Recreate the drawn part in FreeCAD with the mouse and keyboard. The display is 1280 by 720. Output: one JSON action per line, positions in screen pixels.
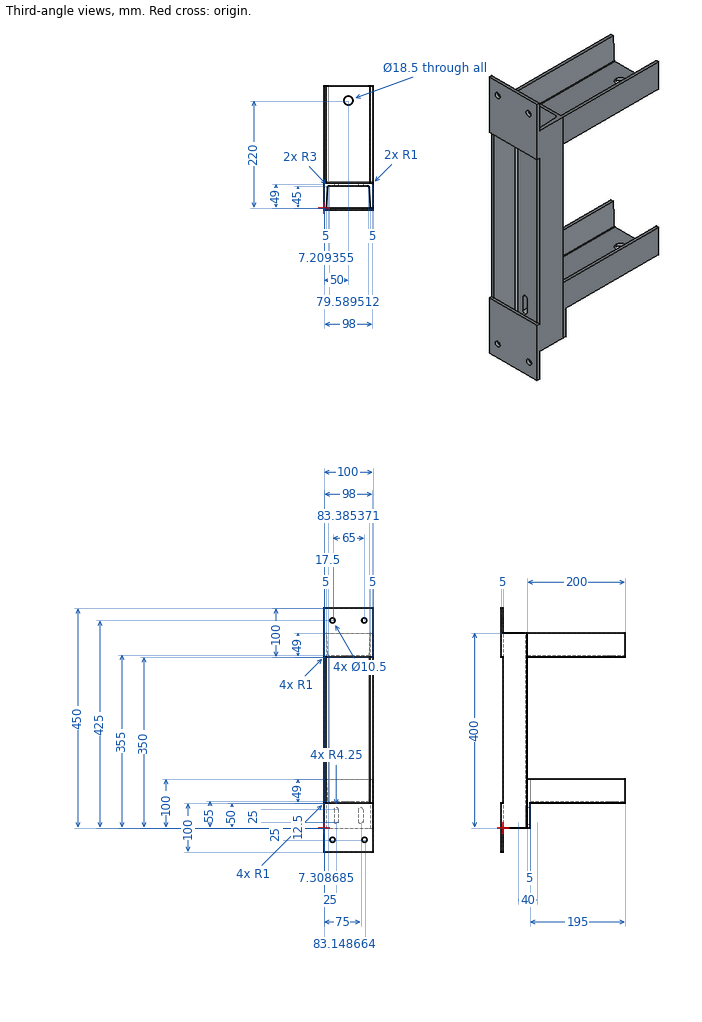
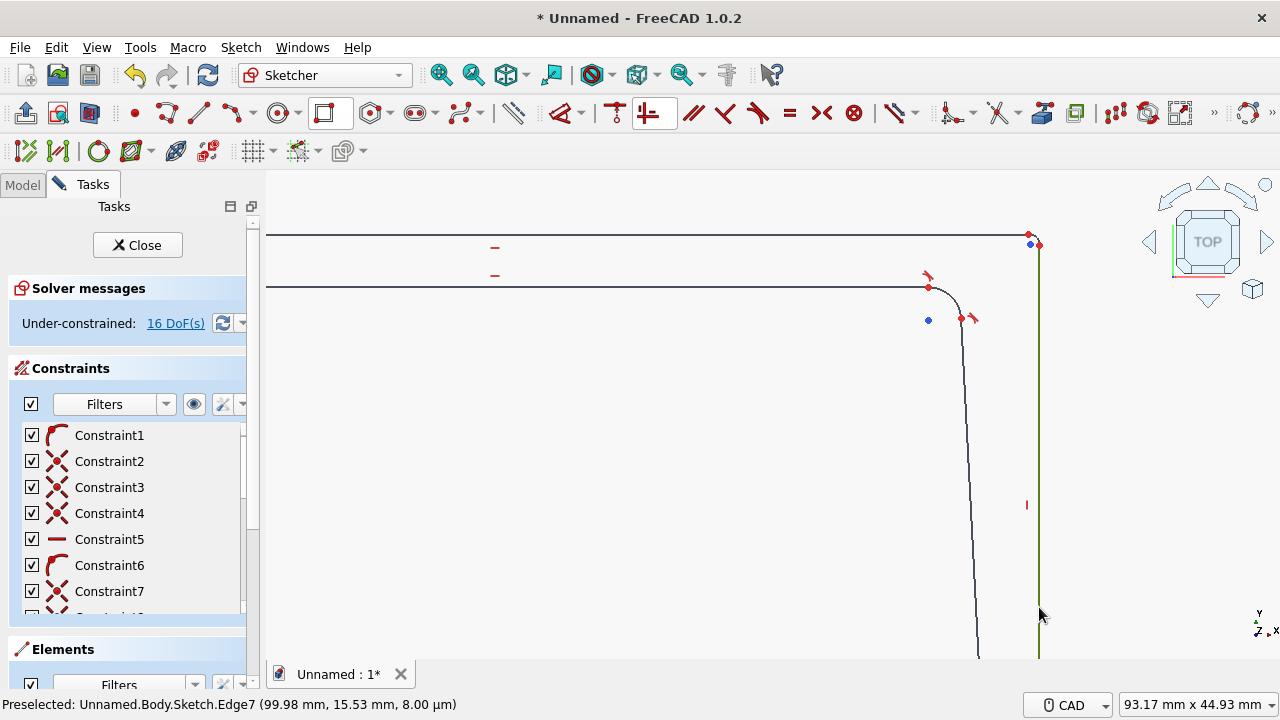
{"action": "scroll", "coordinate": [1037, 237], "scroll_direction": "up", "scroll_amount": 3}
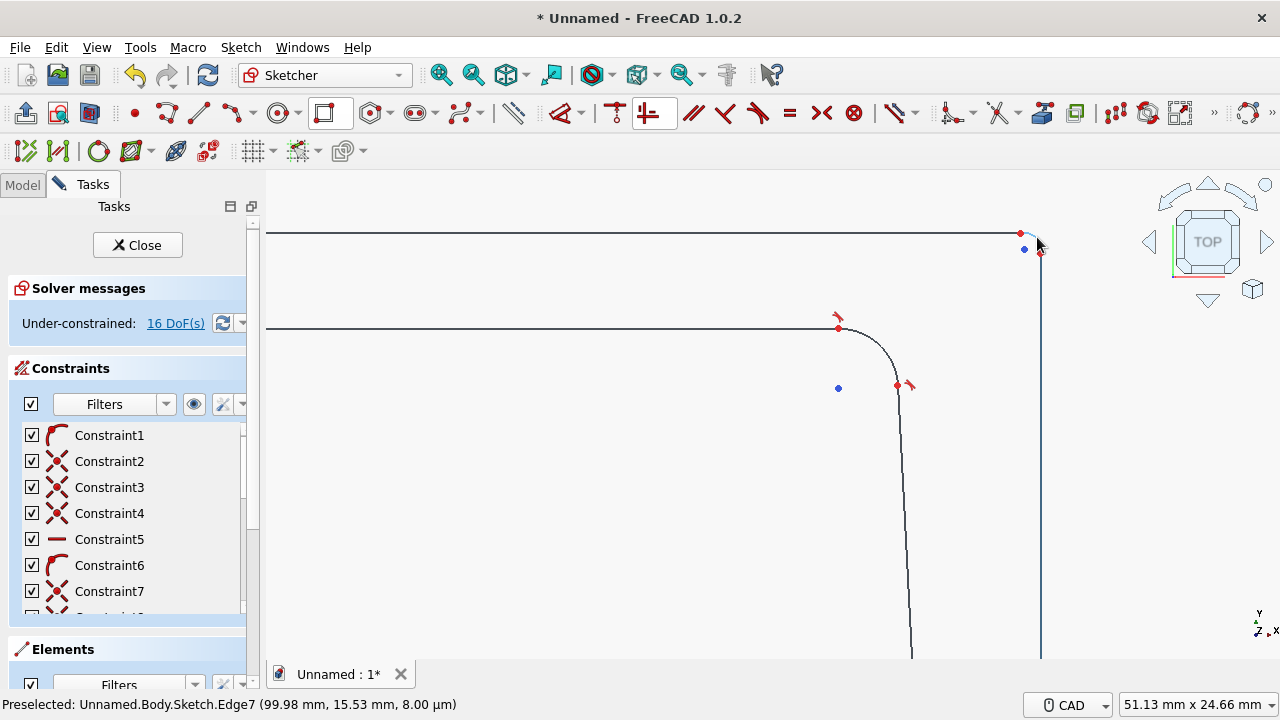
{"action": "left_click", "coordinate": [1036, 238]}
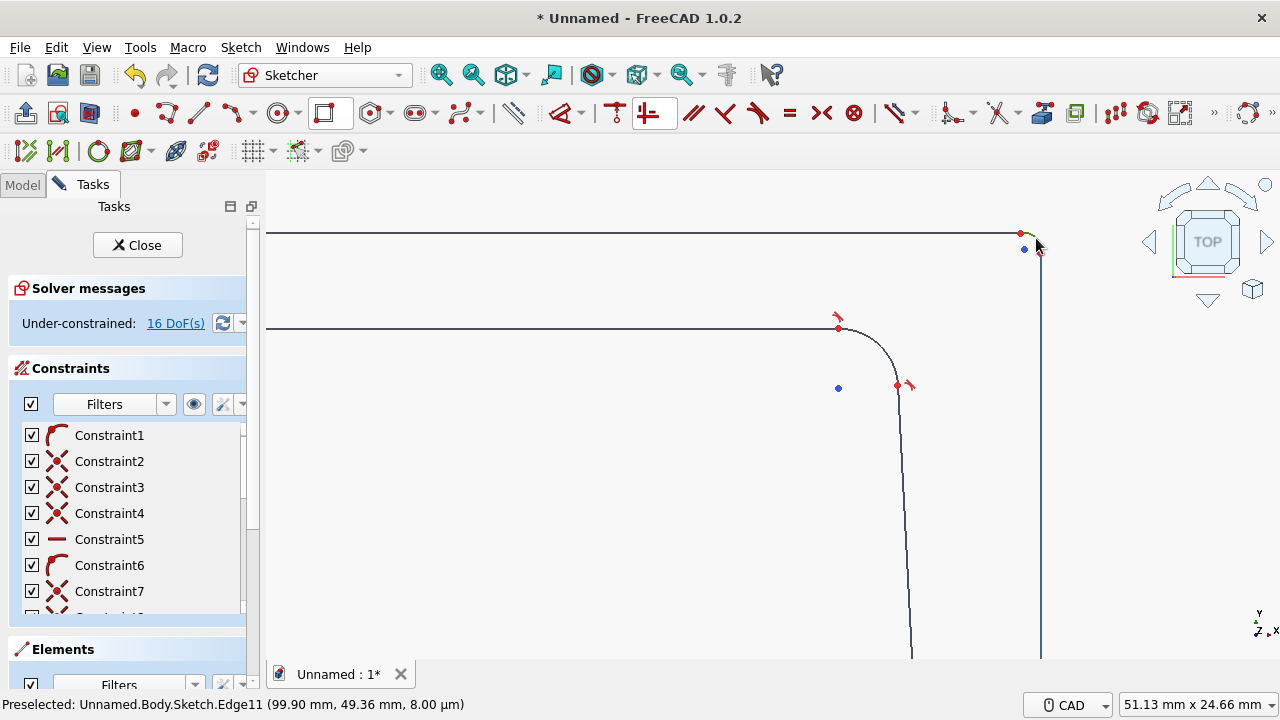
{"action": "left_click", "coordinate": [758, 114]}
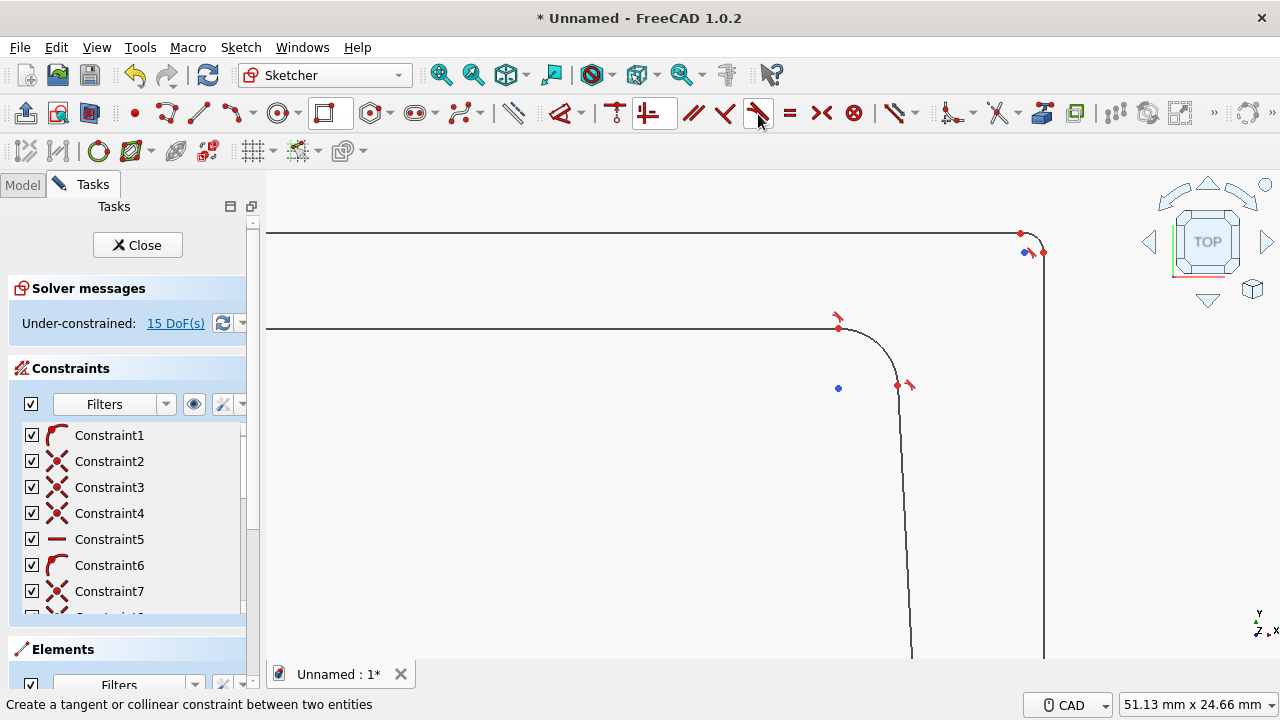
{"action": "left_click", "coordinate": [437, 233]}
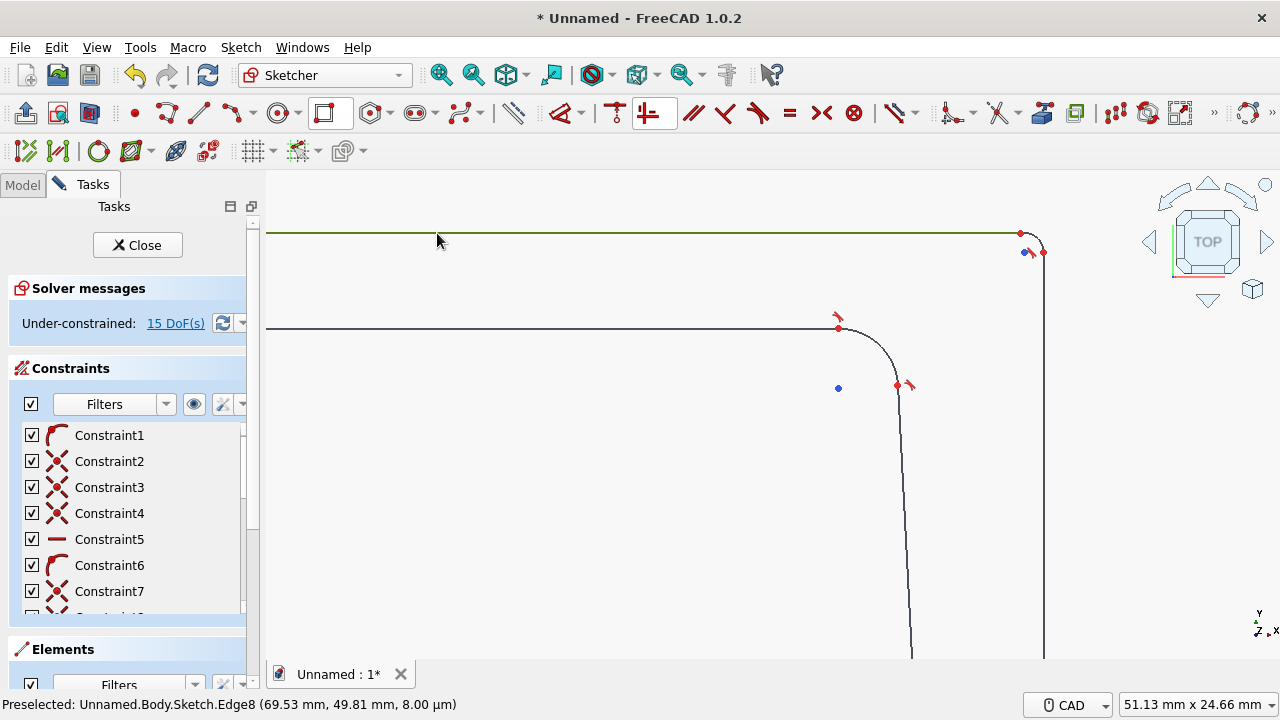
{"action": "scroll", "coordinate": [1041, 242], "scroll_direction": "up", "scroll_amount": 2}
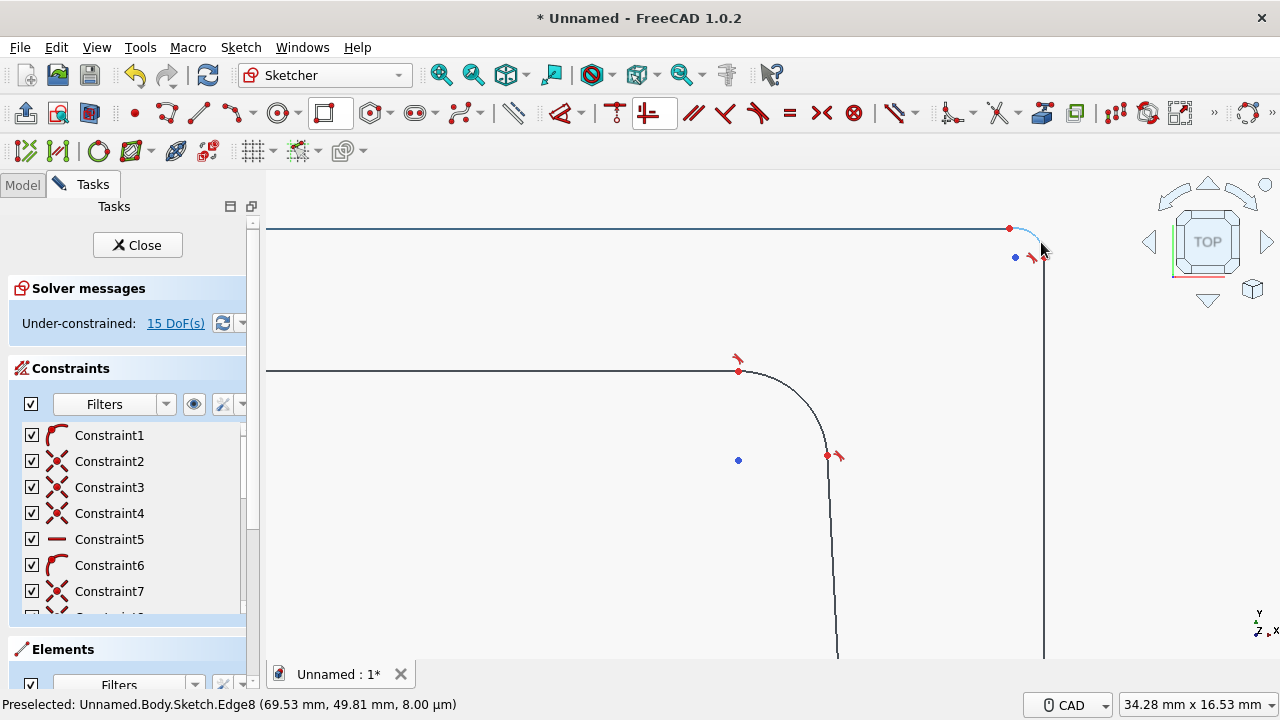
{"action": "left_click", "coordinate": [1040, 243]}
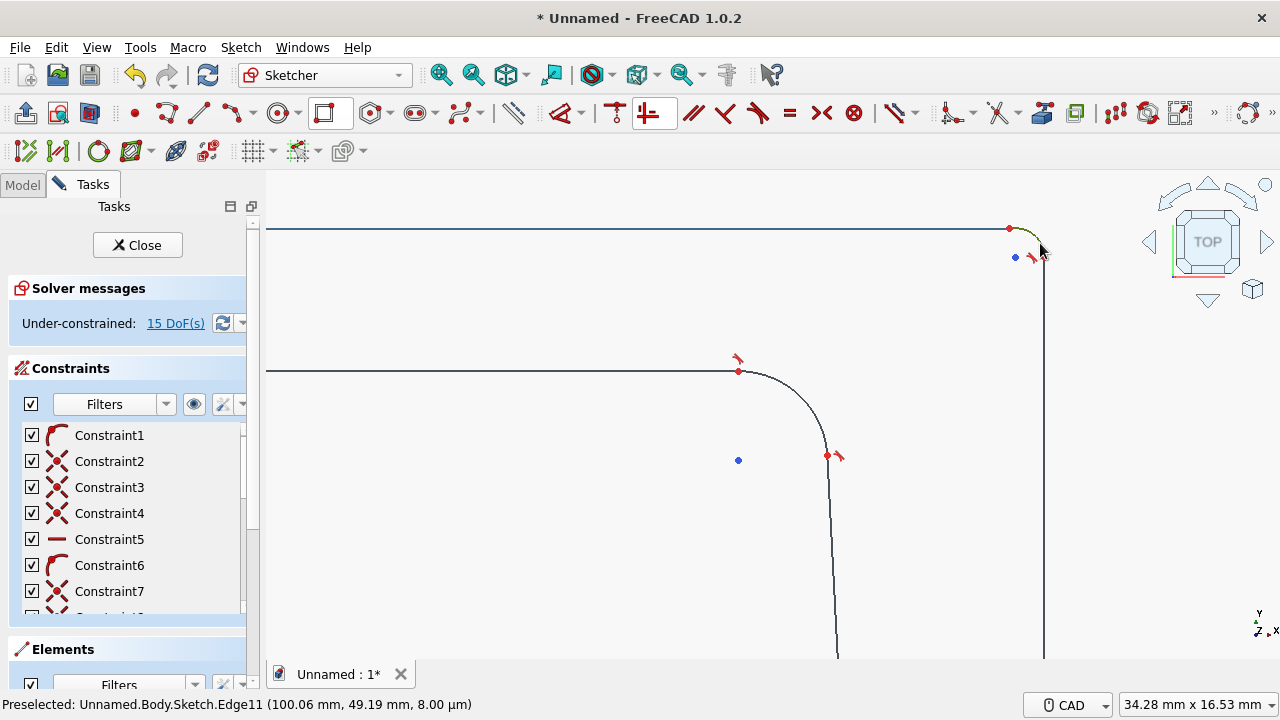
{"action": "left_click", "coordinate": [758, 114]}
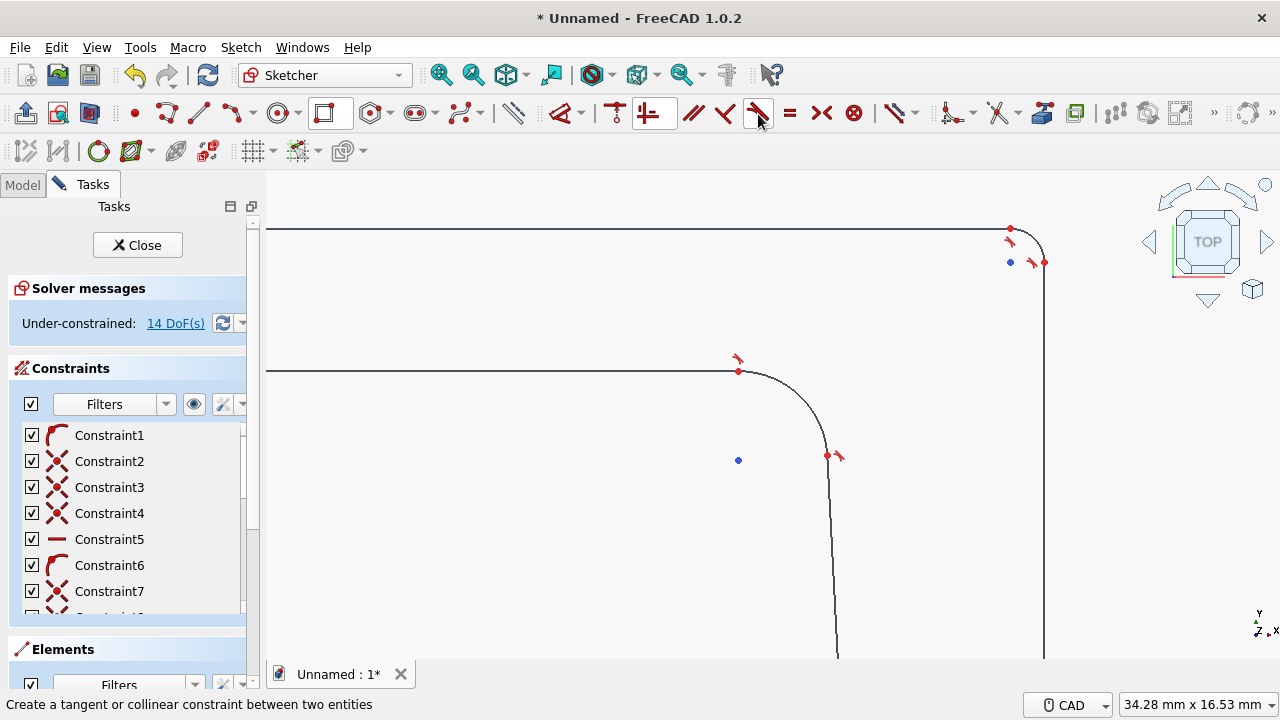
{"action": "scroll", "coordinate": [994, 276], "scroll_direction": "down", "scroll_amount": 8}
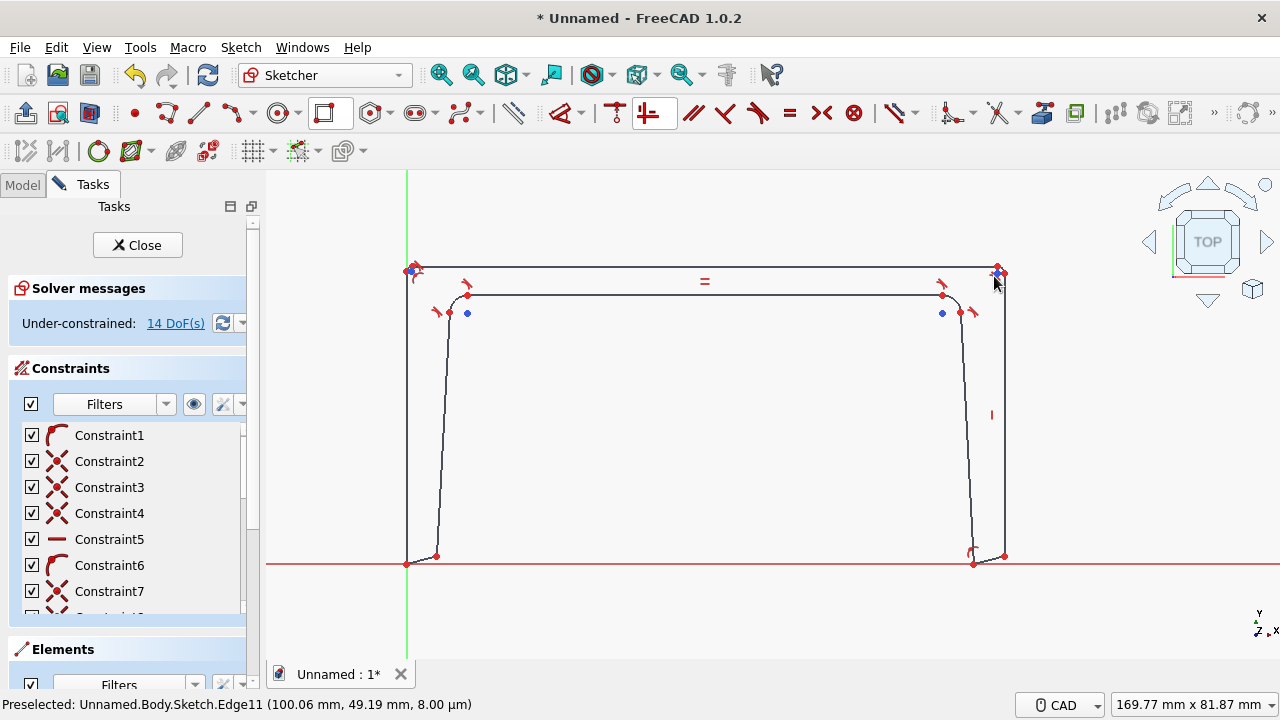
{"action": "left_click", "coordinate": [881, 267]}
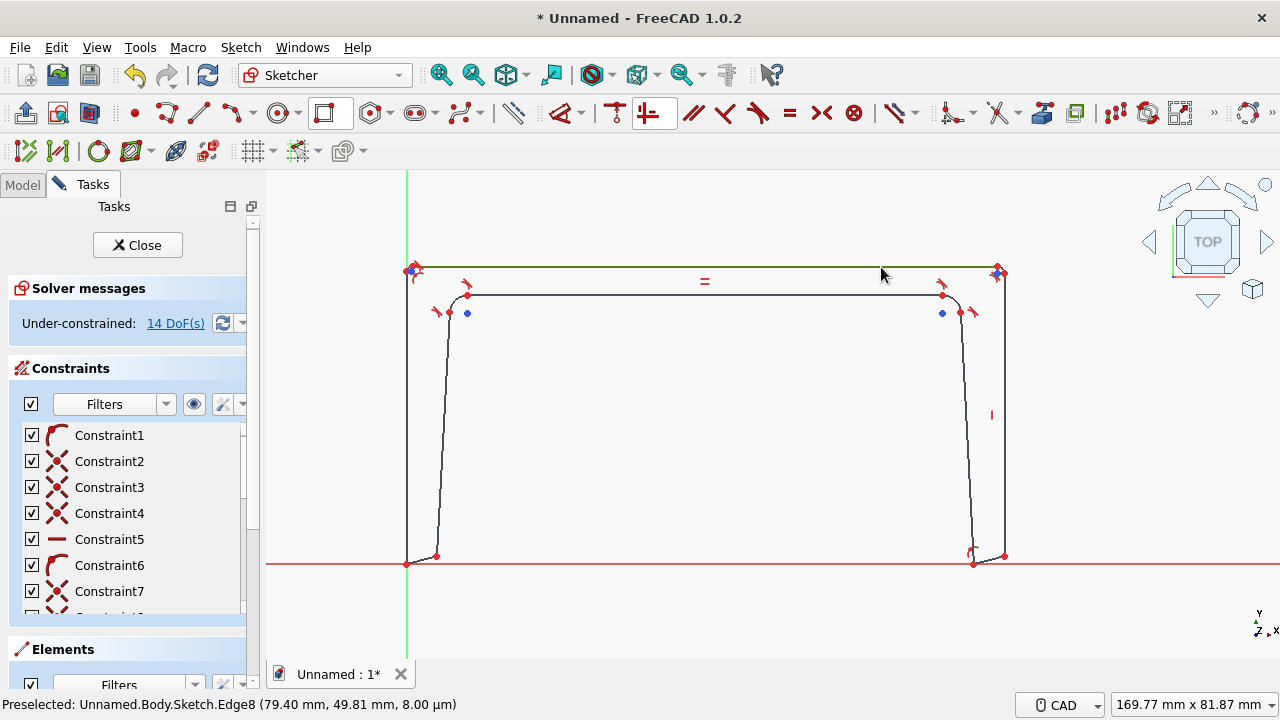
{"action": "scroll", "coordinate": [409, 268], "scroll_direction": "up", "scroll_amount": 6}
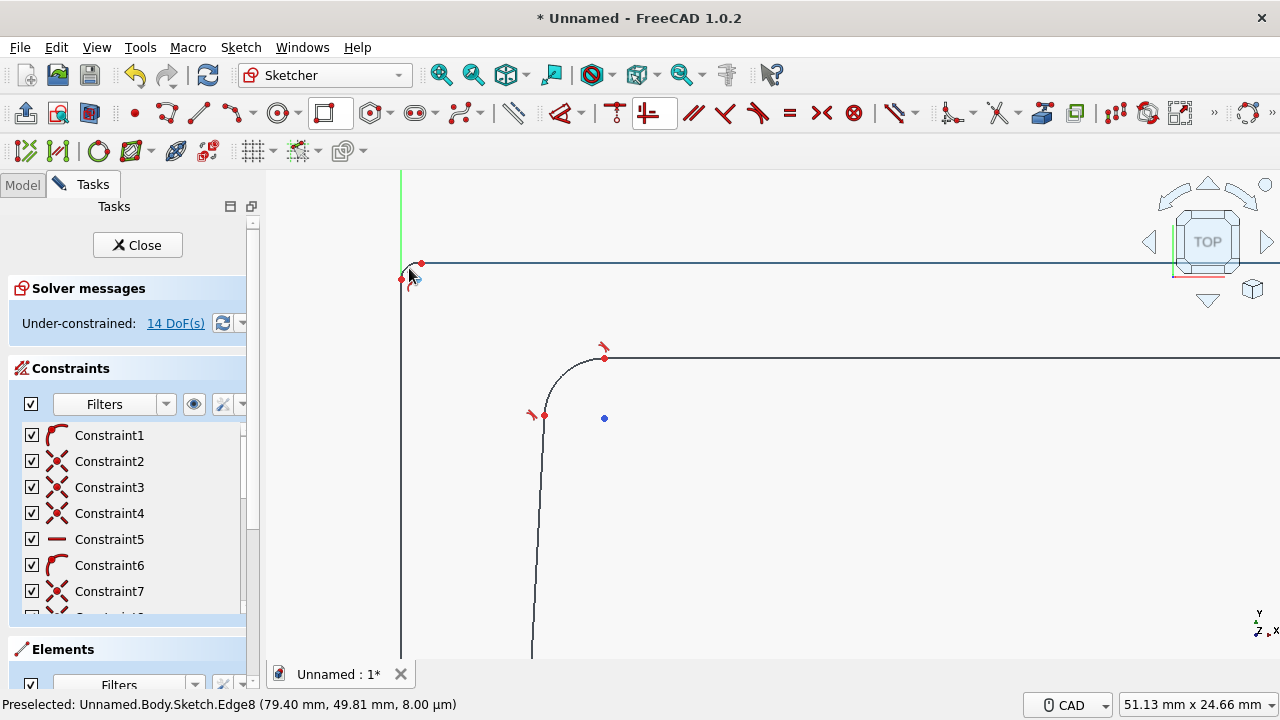
{"action": "left_click", "coordinate": [407, 267]}